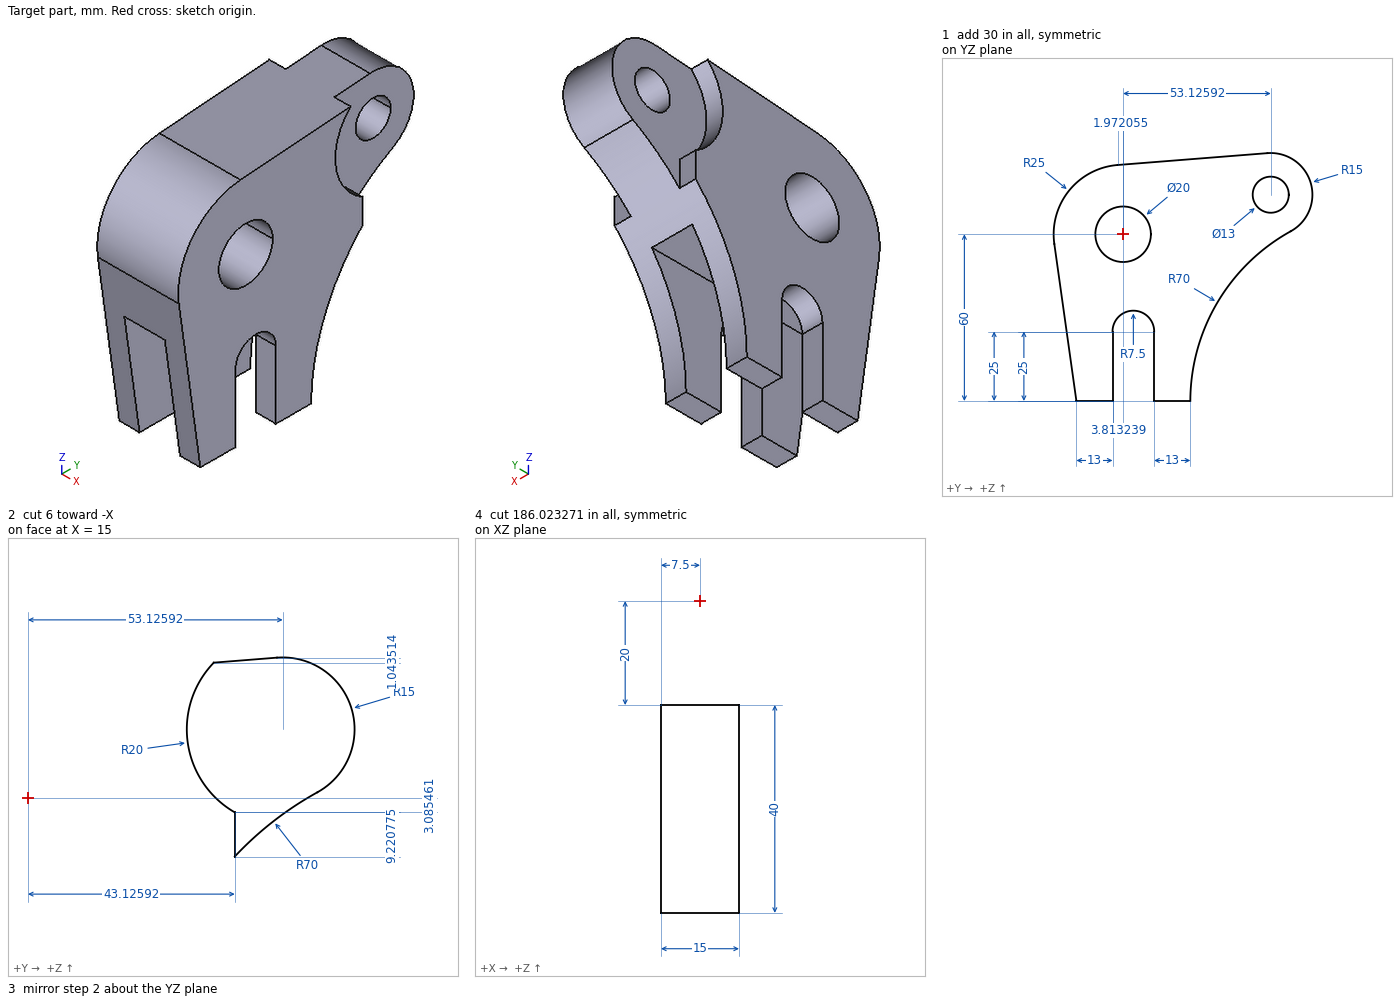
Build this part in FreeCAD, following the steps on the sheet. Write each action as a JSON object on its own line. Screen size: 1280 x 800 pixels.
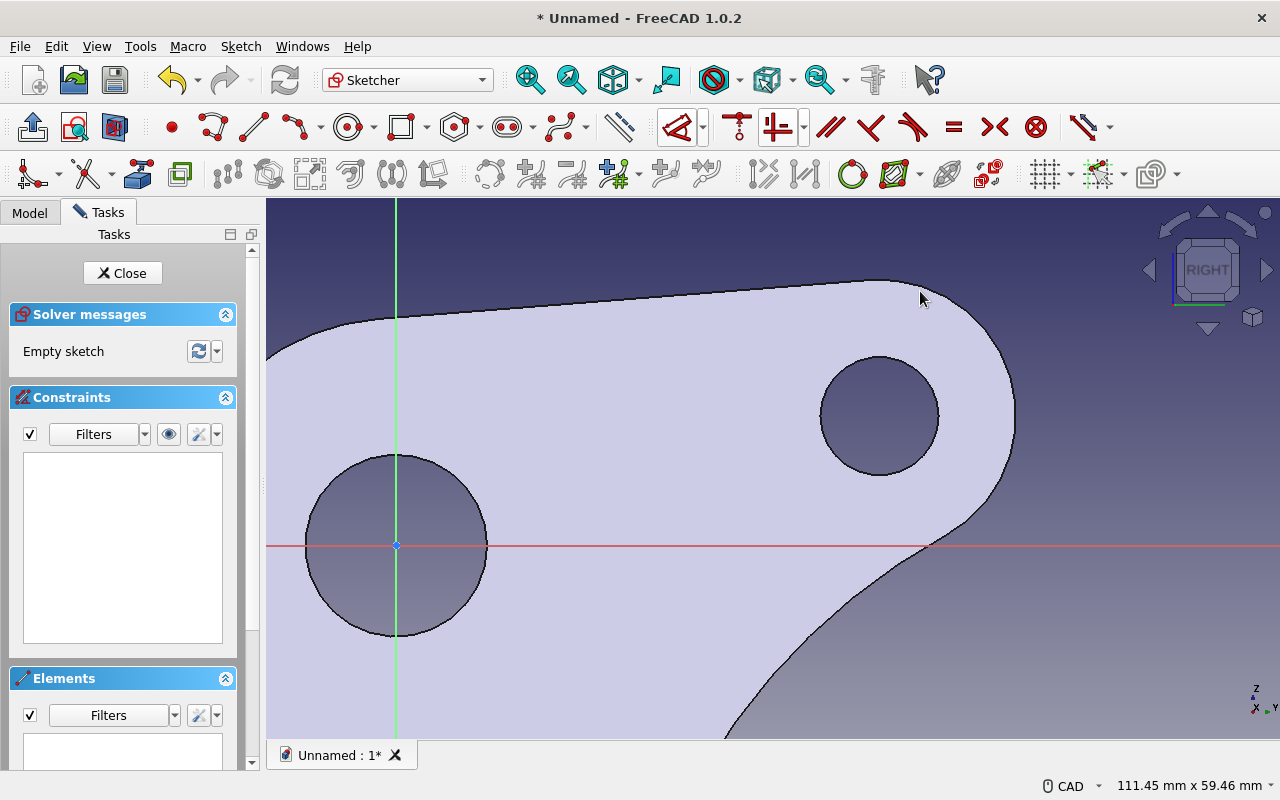
{"action": "left_click", "coordinate": [254, 128]}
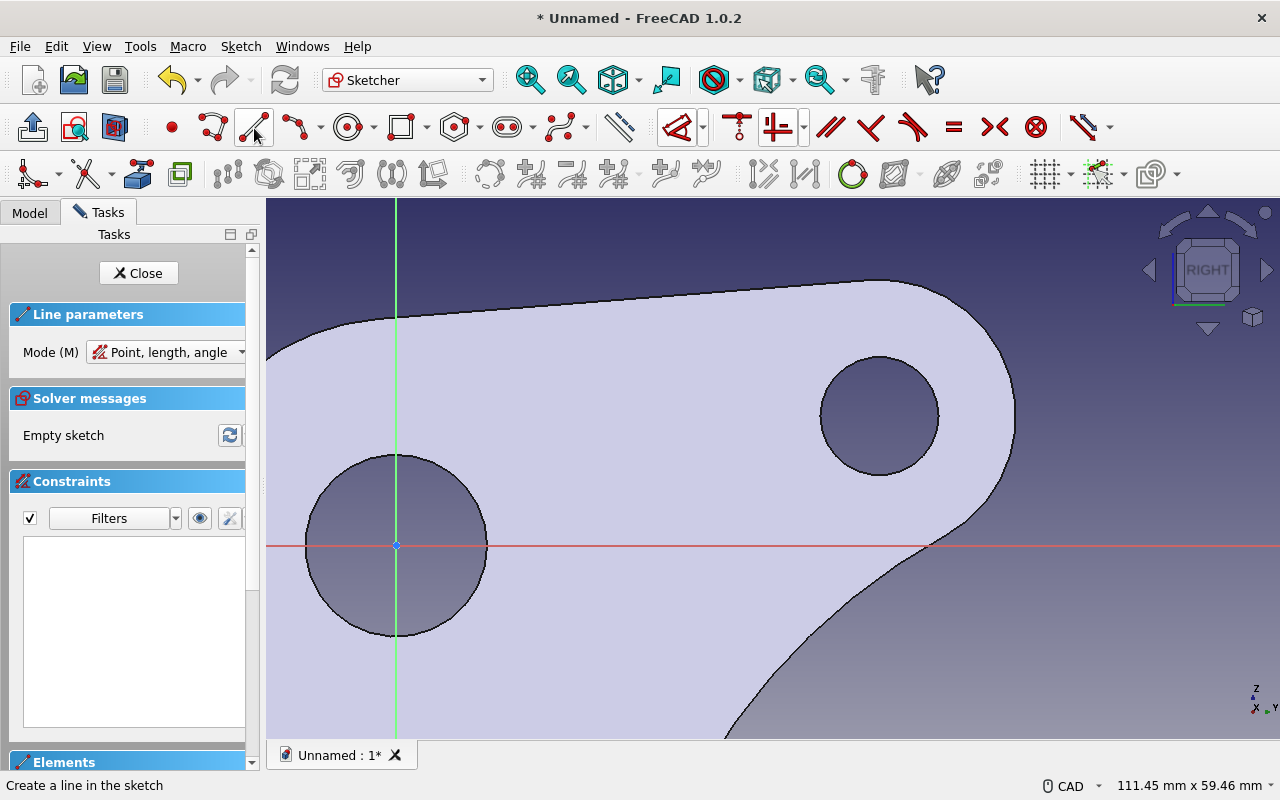
{"action": "left_click", "coordinate": [789, 574]}
{"action": "left_click", "coordinate": [789, 658]}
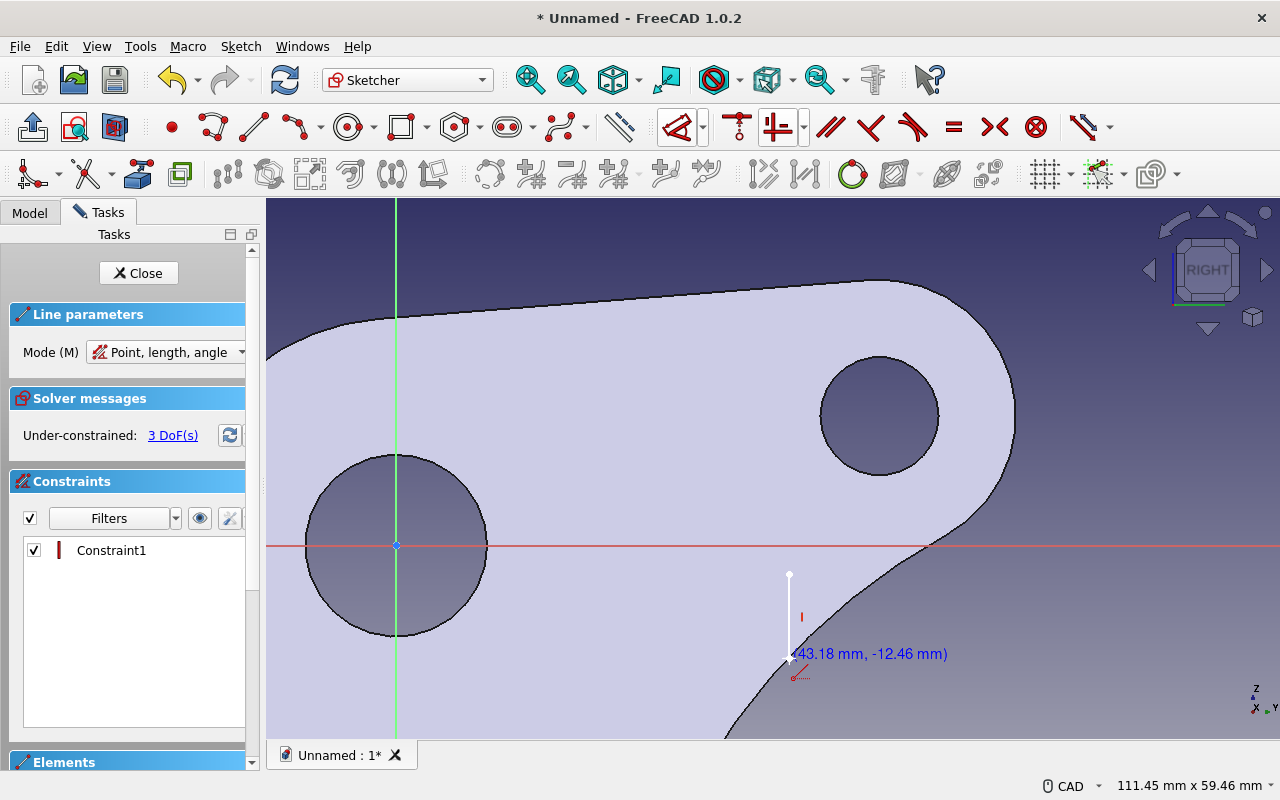
{"action": "left_click", "coordinate": [869, 280]}
{"action": "left_click", "coordinate": [749, 290]}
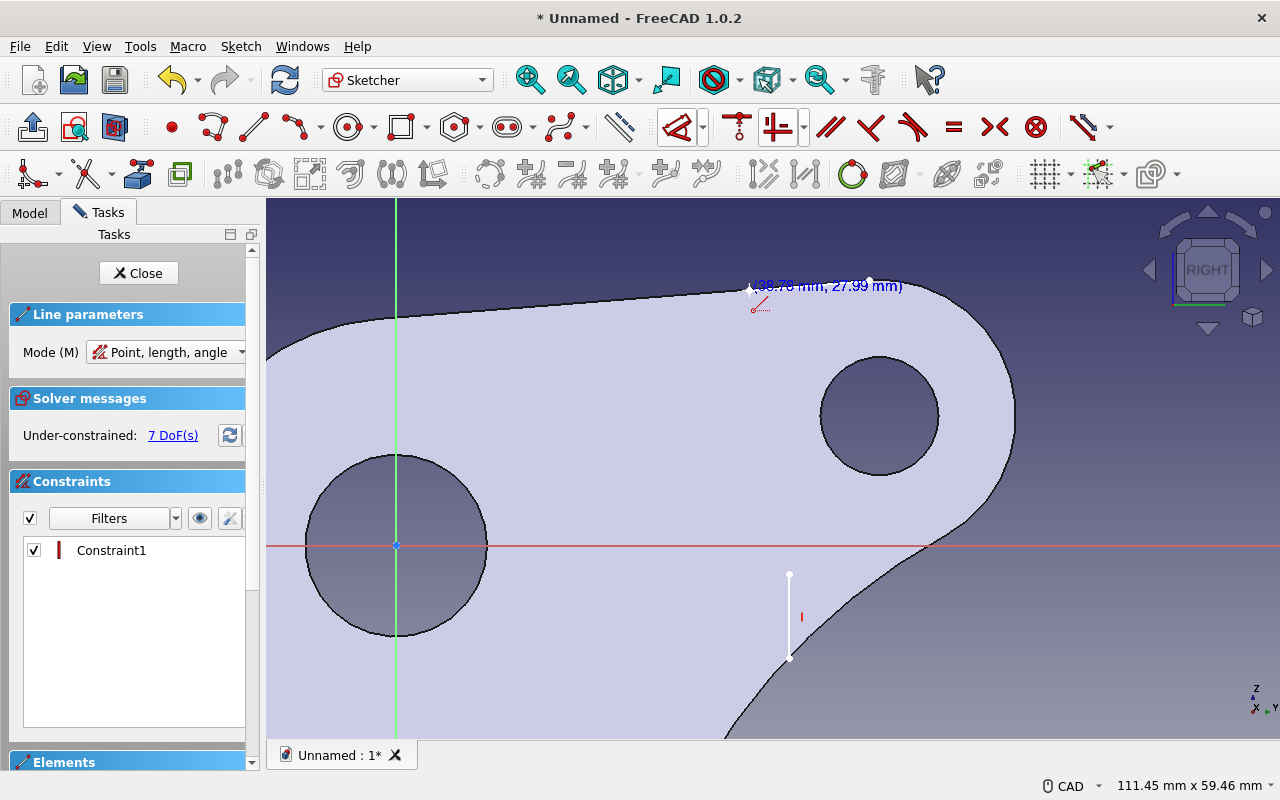
{"action": "left_click", "coordinate": [294, 128]}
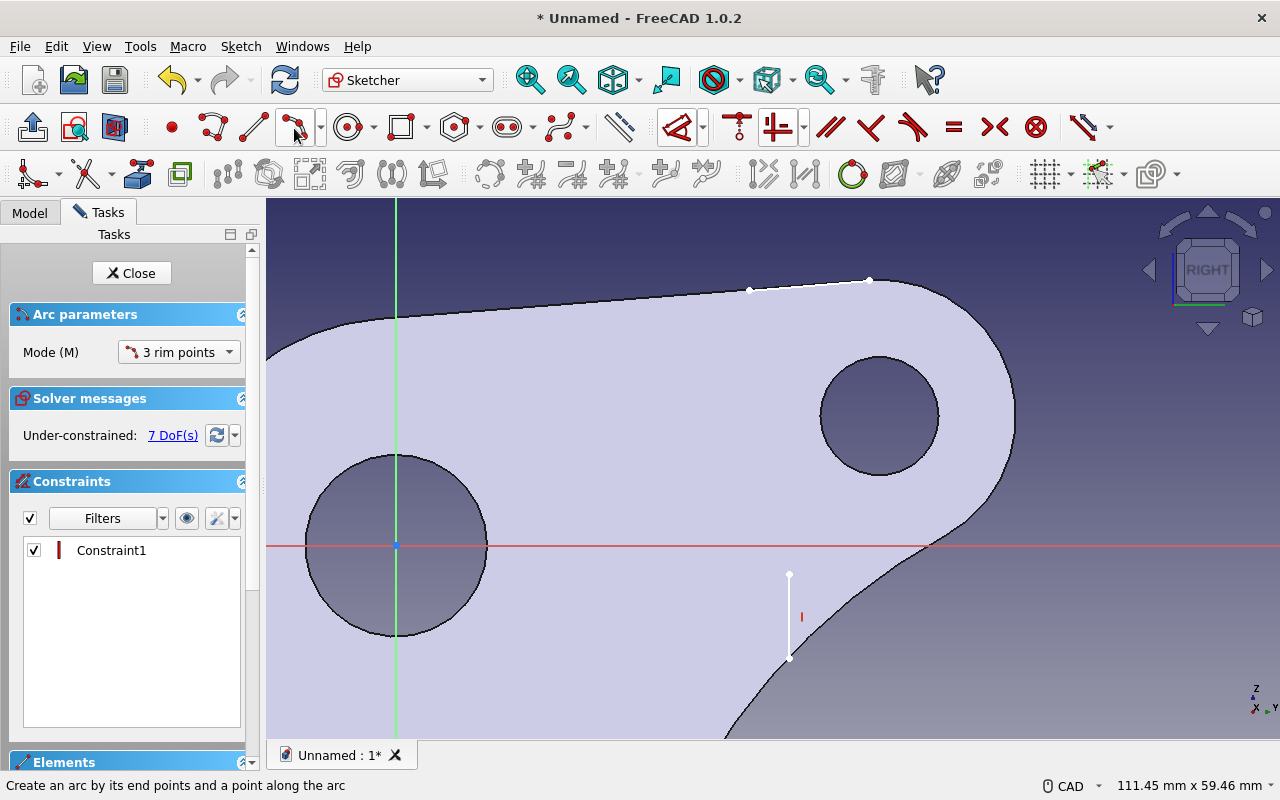
{"action": "left_click", "coordinate": [789, 659]}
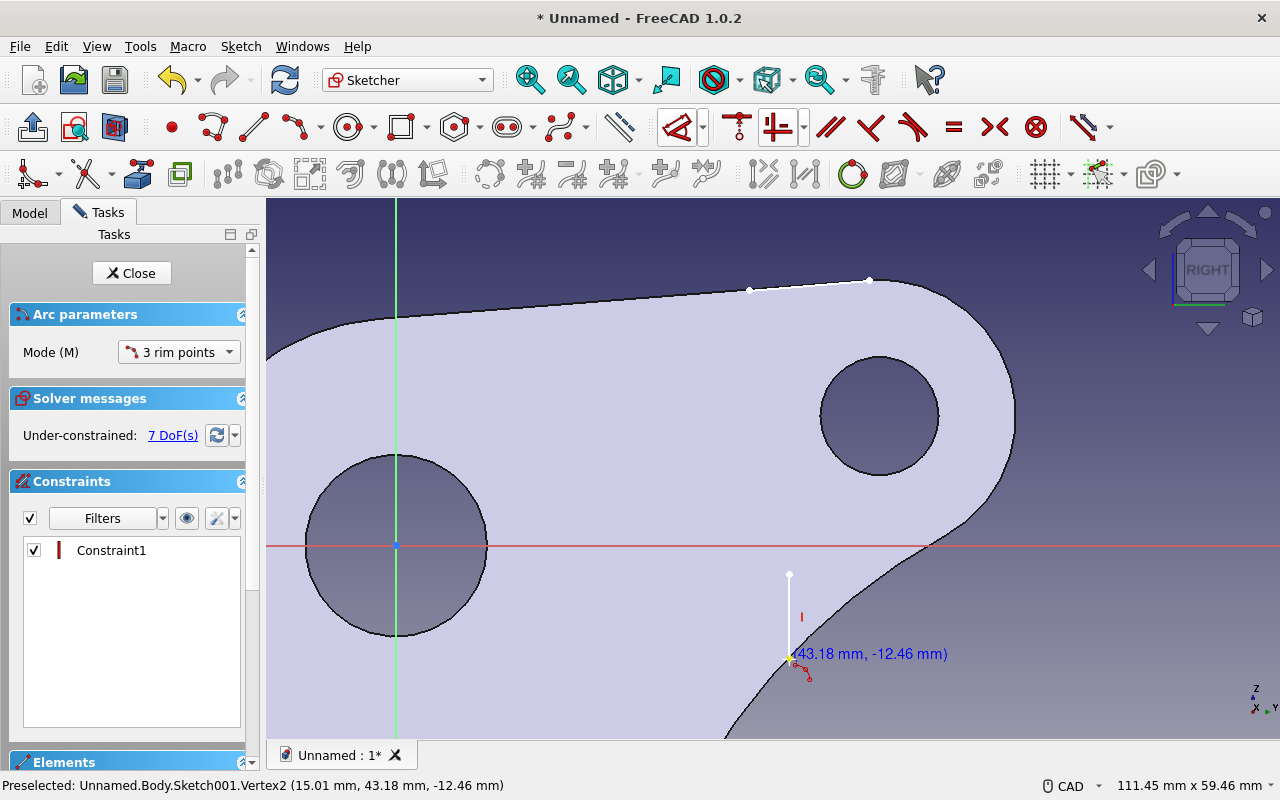
{"action": "scroll", "coordinate": [945, 536], "scroll_direction": "up", "scroll_amount": 3}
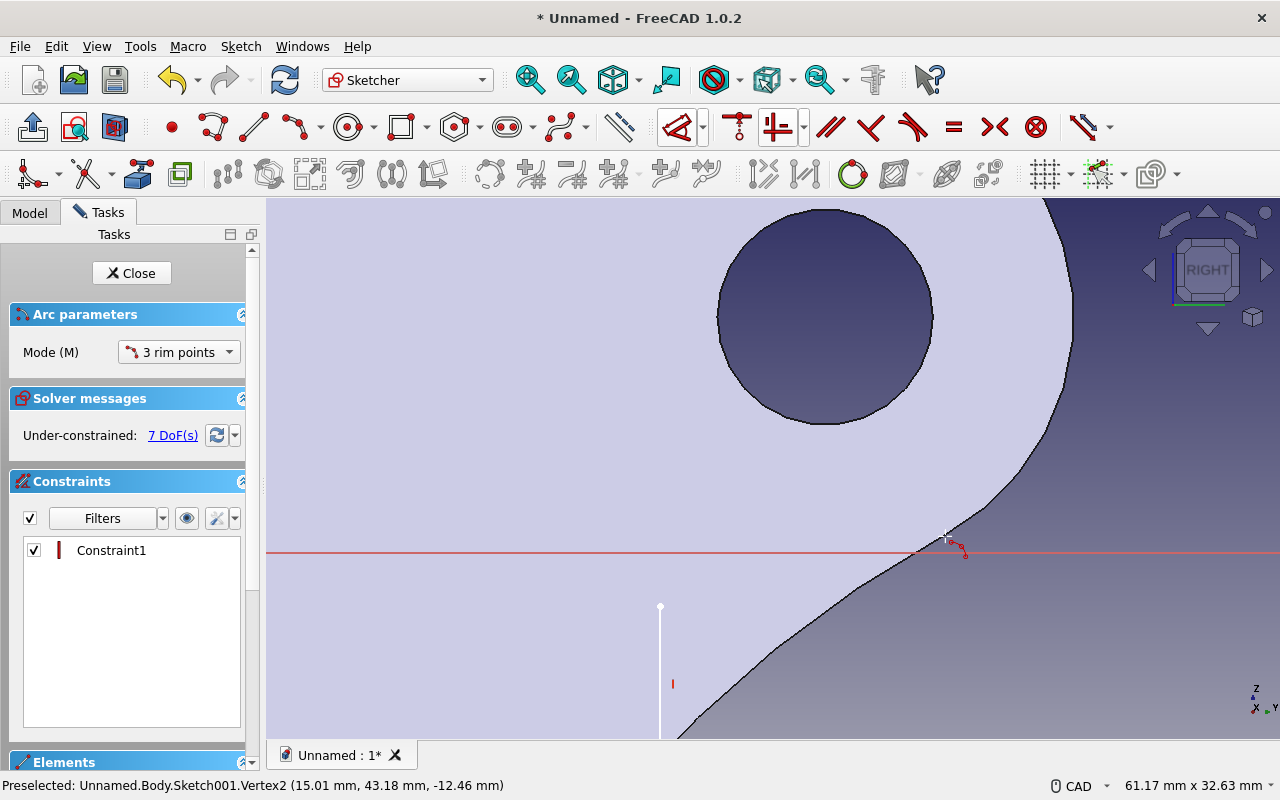
{"action": "left_click", "coordinate": [945, 535]}
{"action": "left_click", "coordinate": [794, 635]}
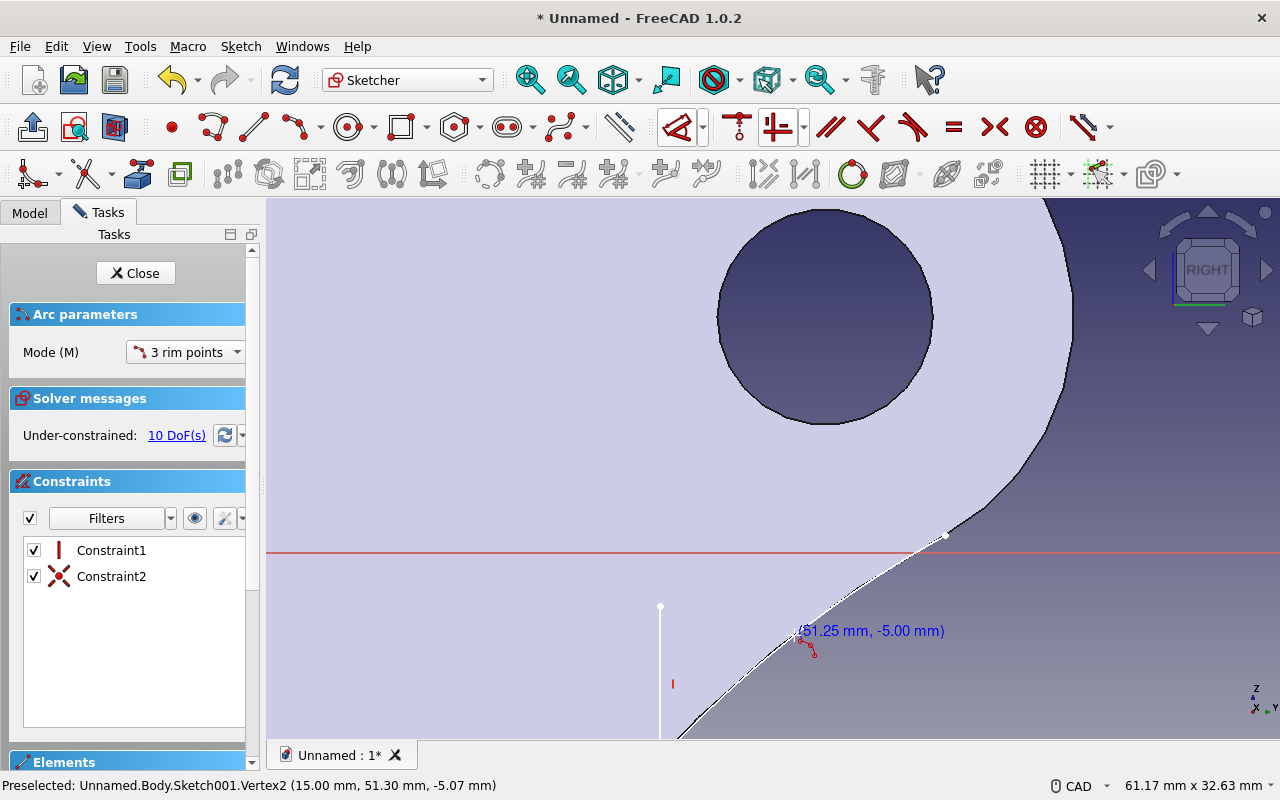
{"action": "left_click", "coordinate": [945, 536]}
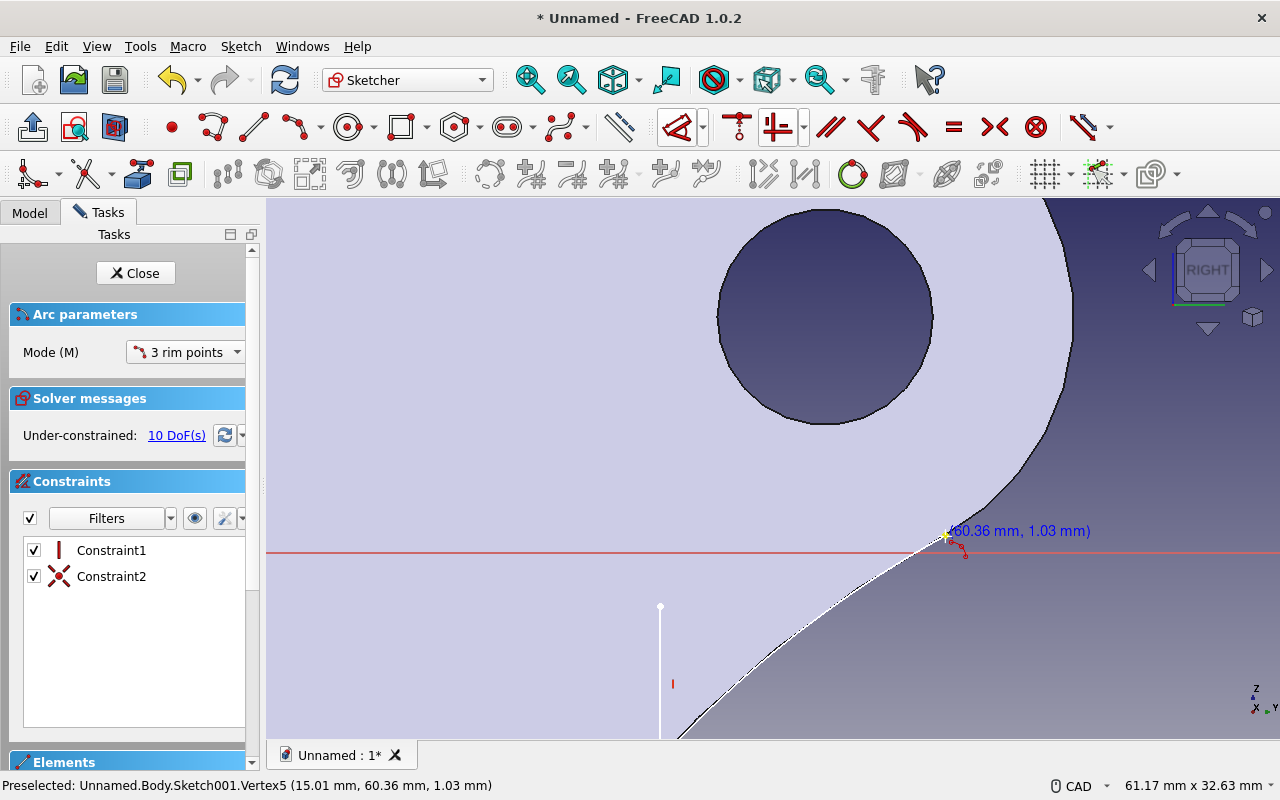
{"action": "scroll", "coordinate": [949, 536], "scroll_direction": "down", "scroll_amount": 3}